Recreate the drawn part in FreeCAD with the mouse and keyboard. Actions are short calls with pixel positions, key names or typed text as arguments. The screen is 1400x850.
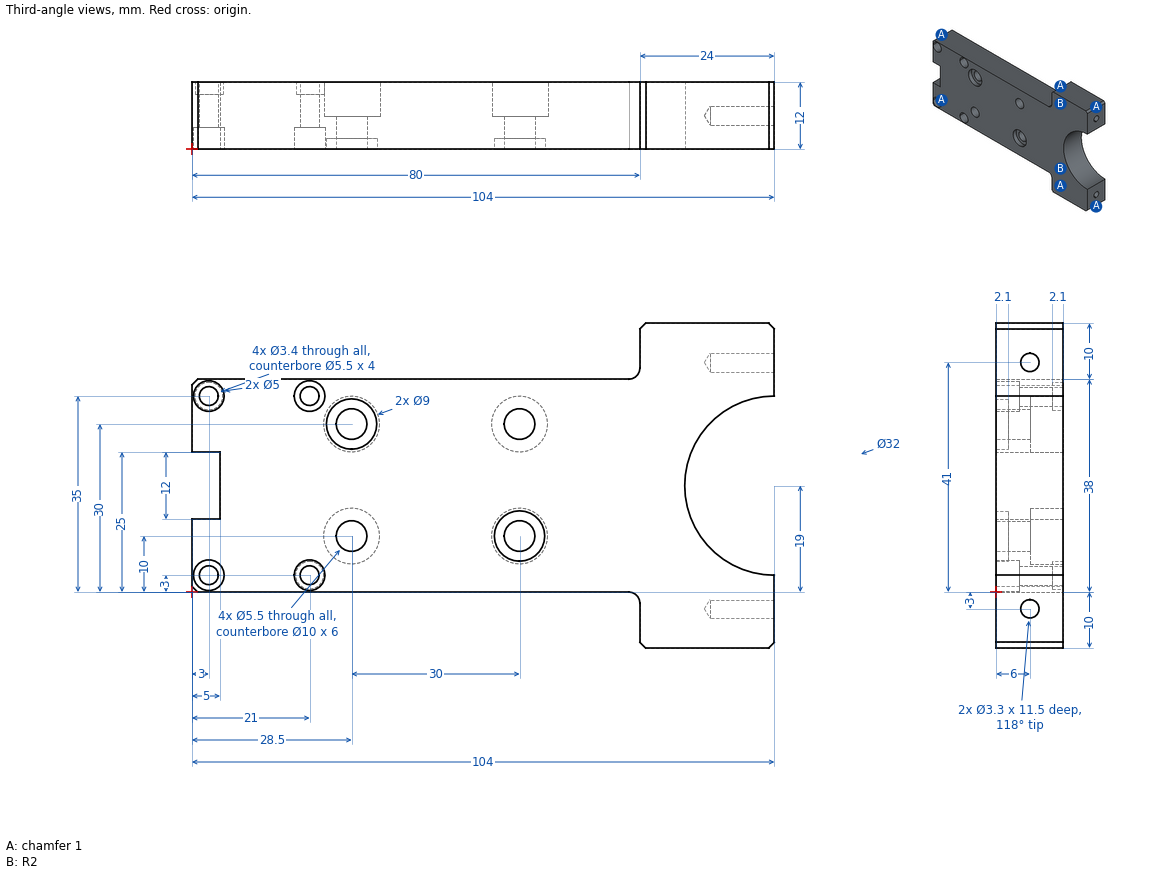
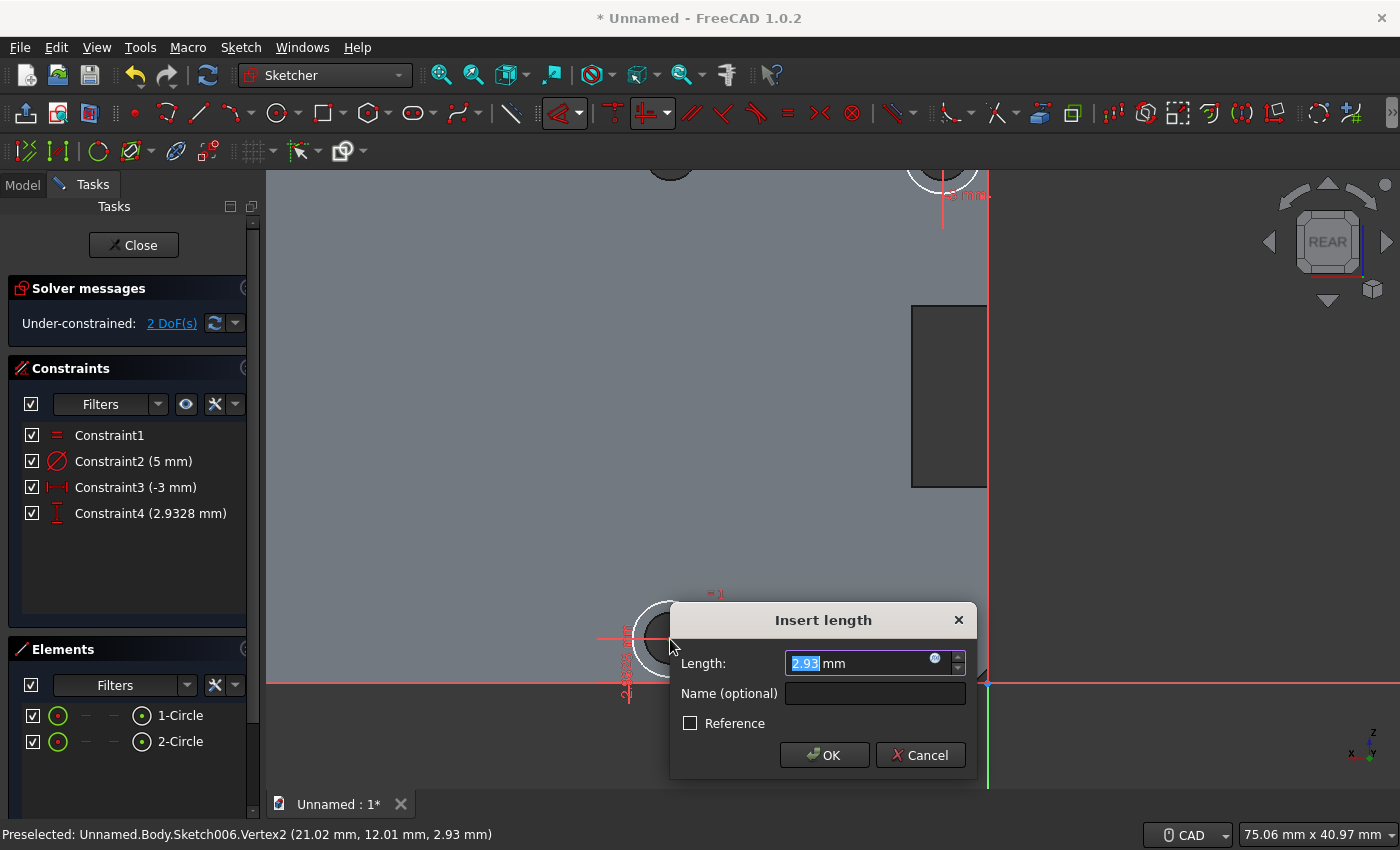
text(3)
key(Return)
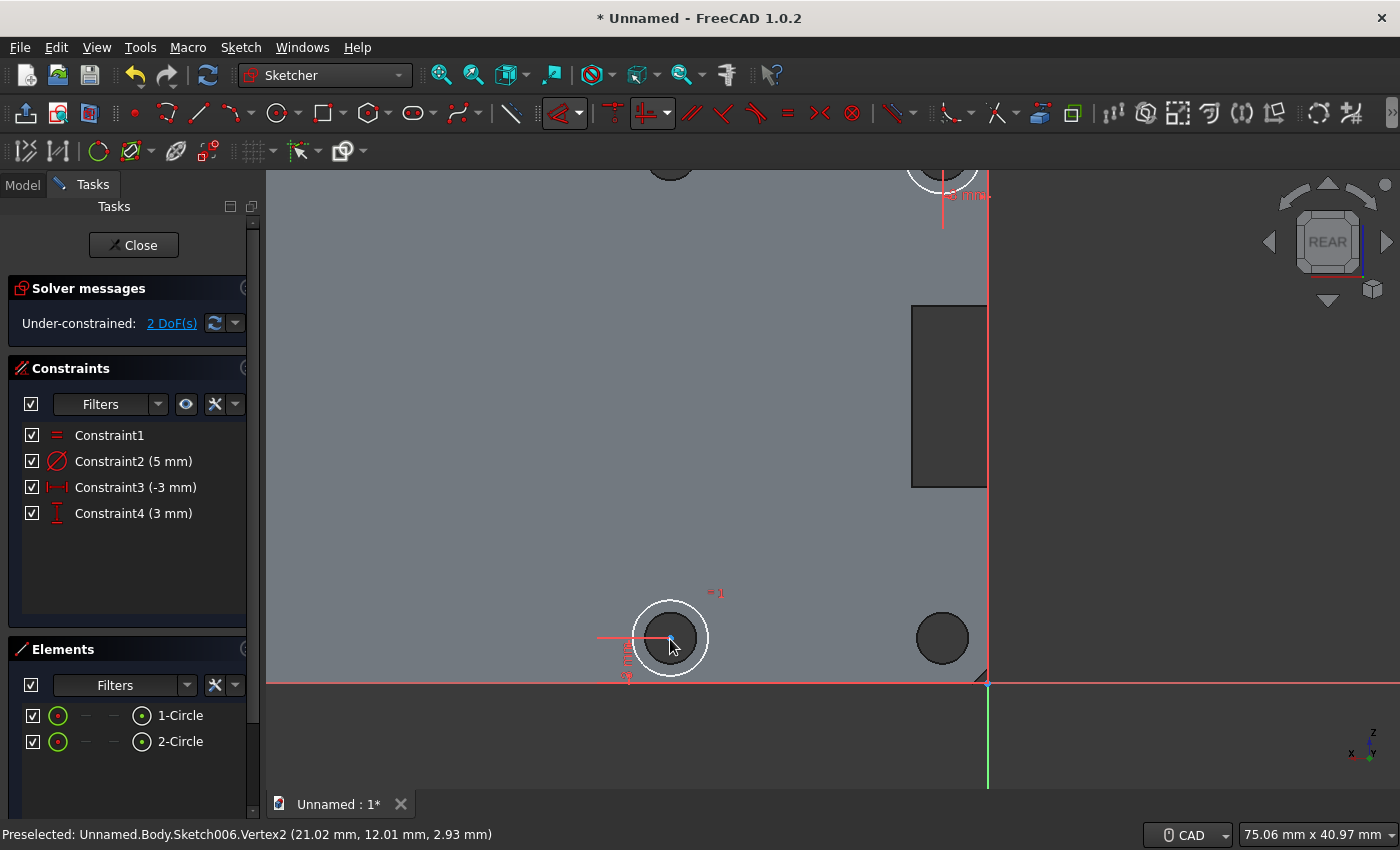
scroll(671, 641, down, 2)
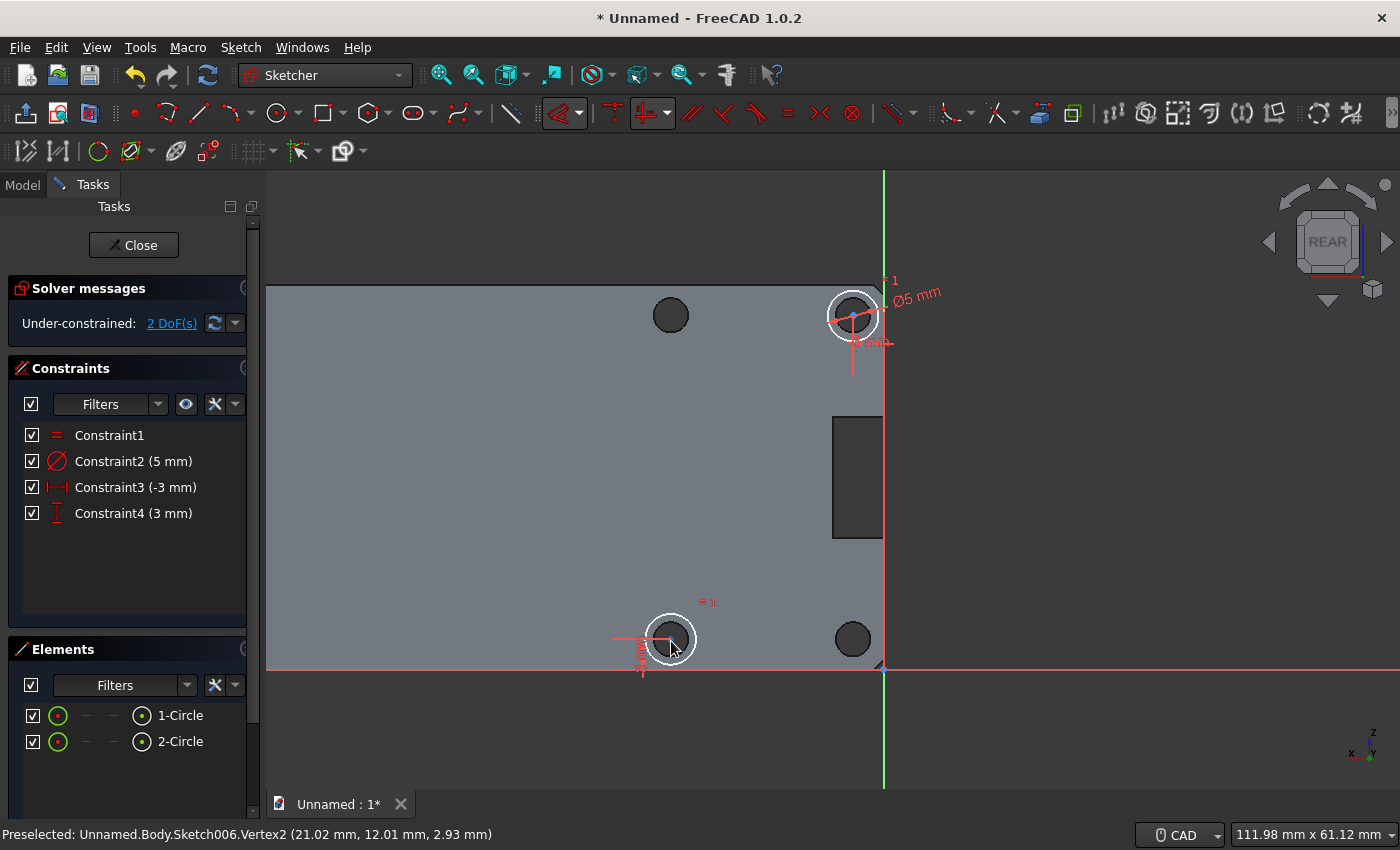
click(853, 316)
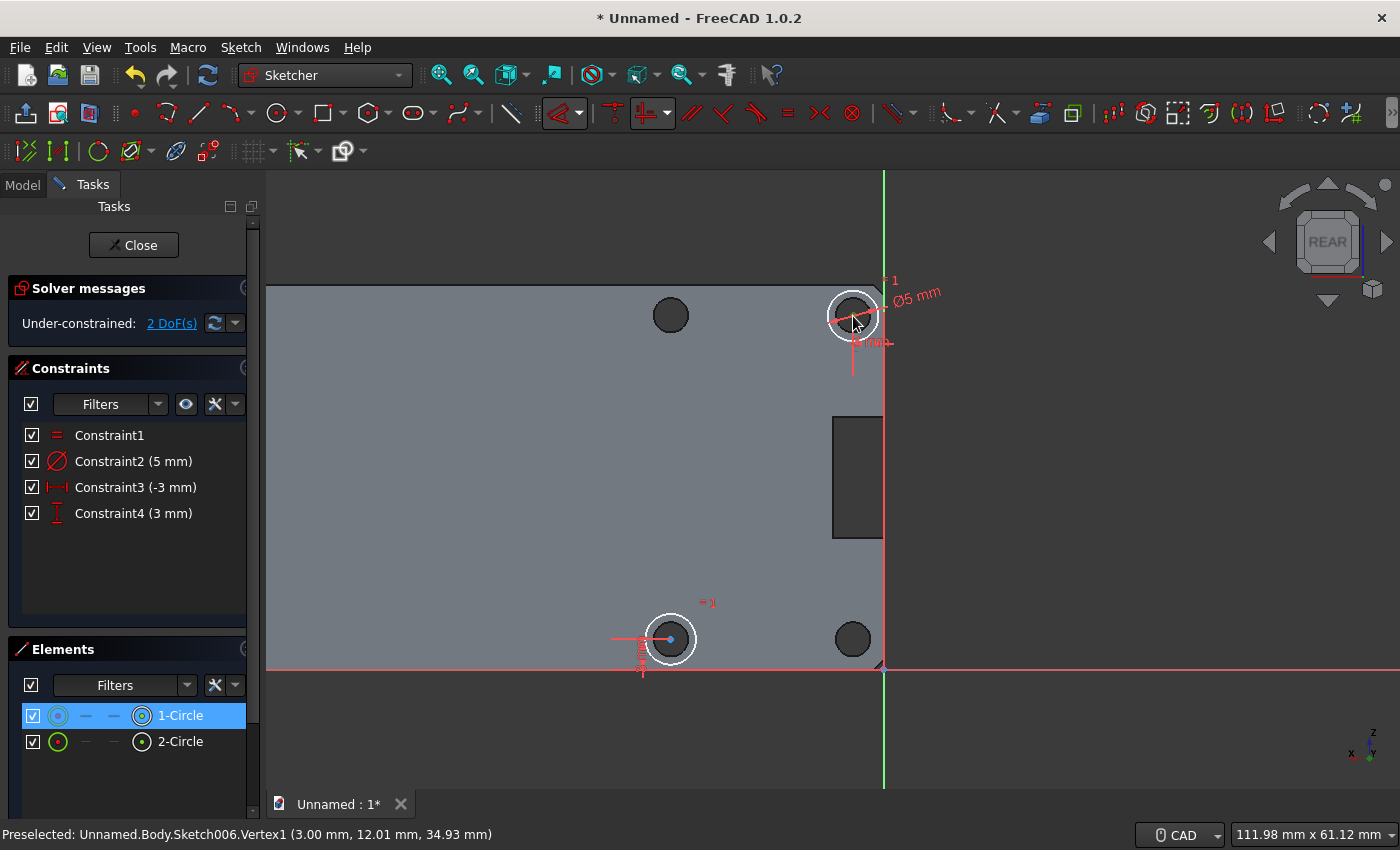
key(i)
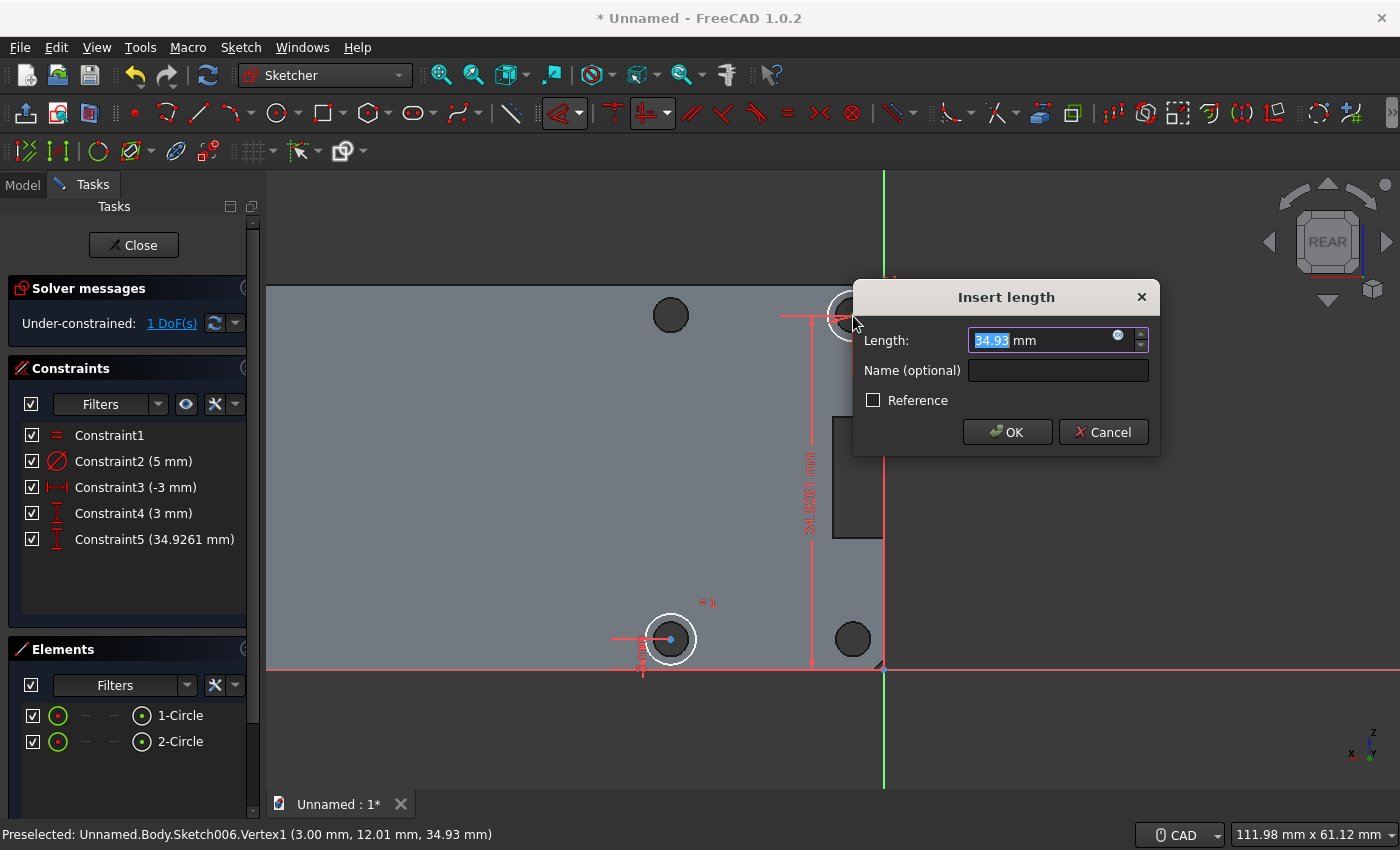
text(35)
key(Return)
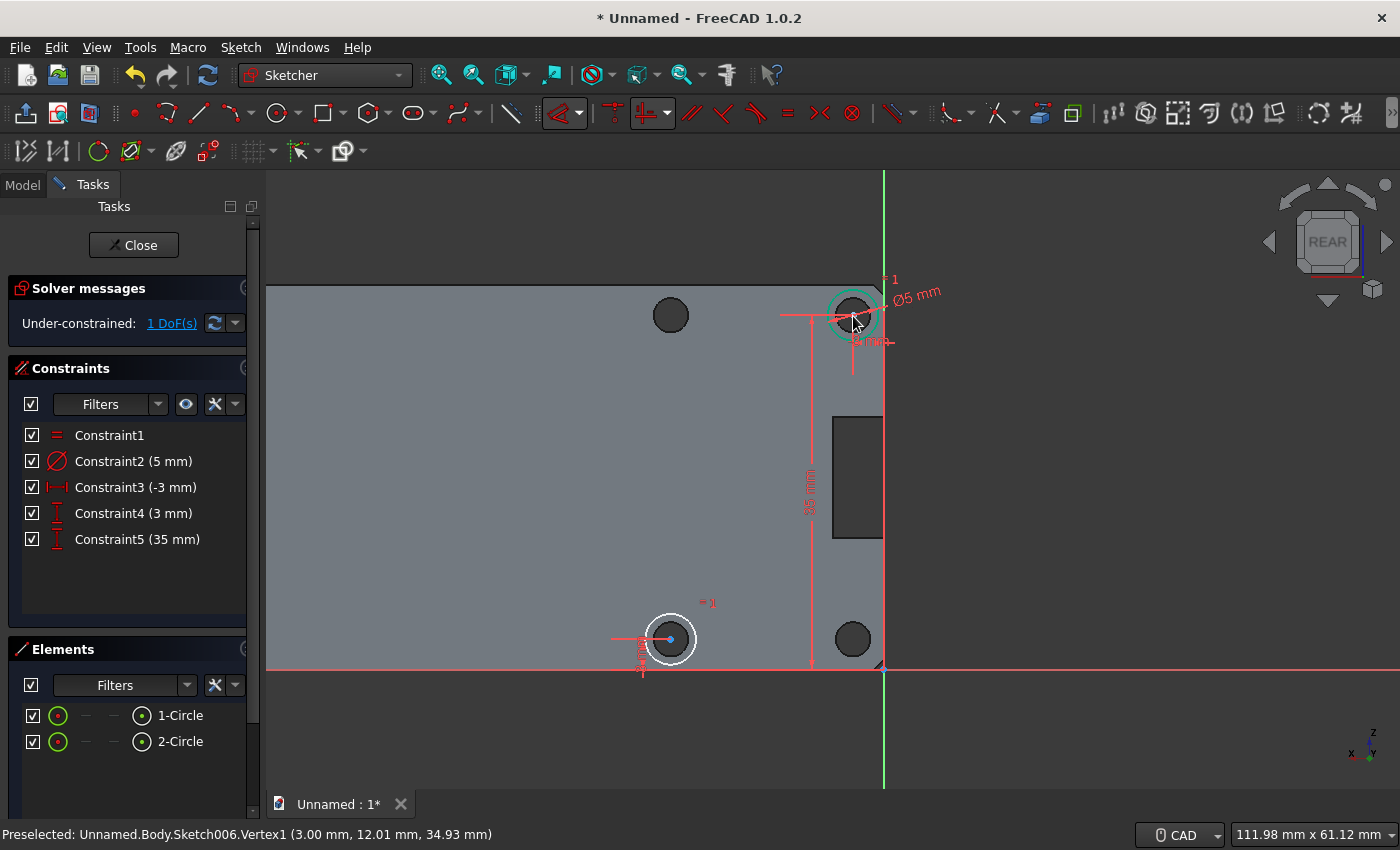
click(671, 639)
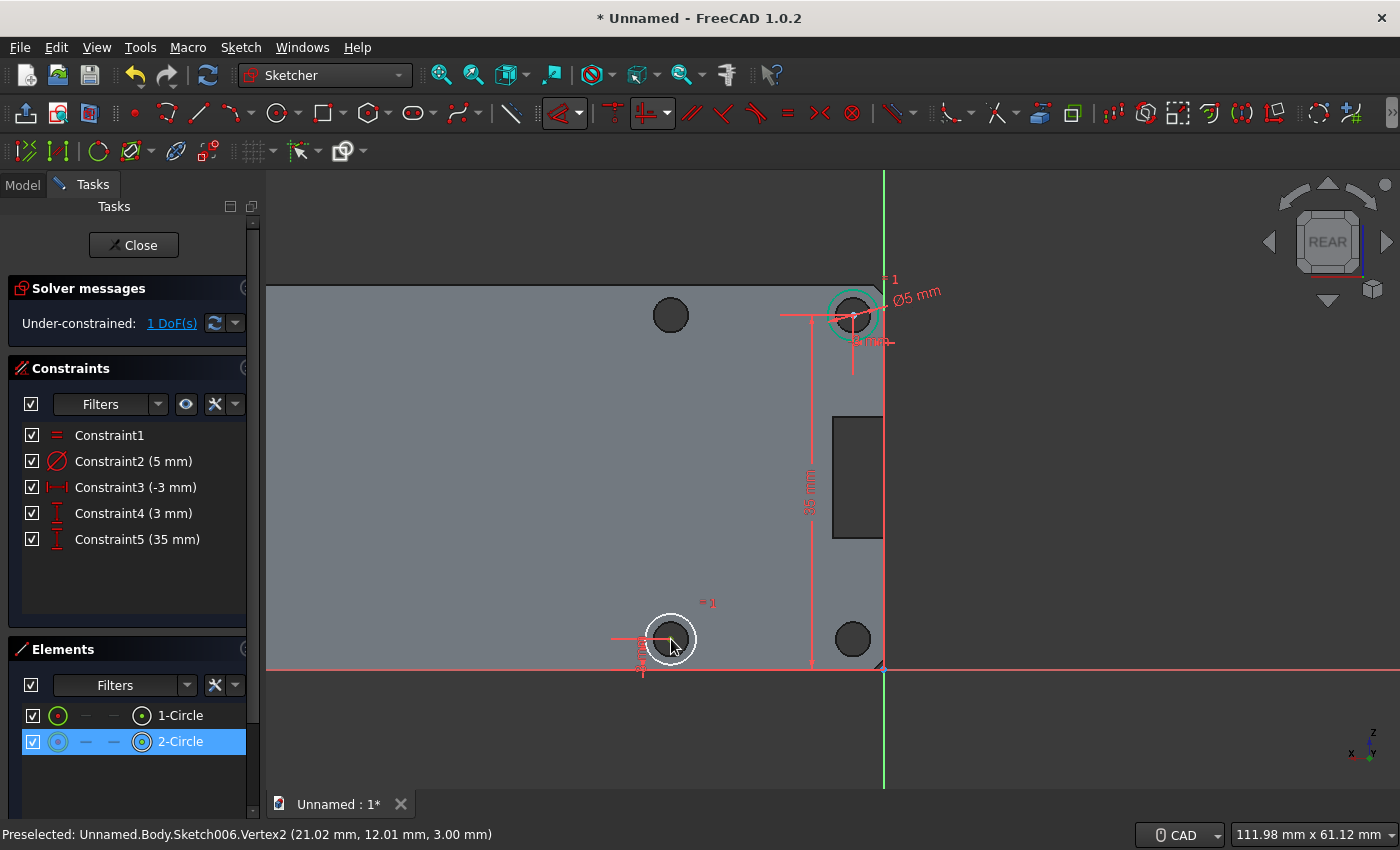
click(582, 114)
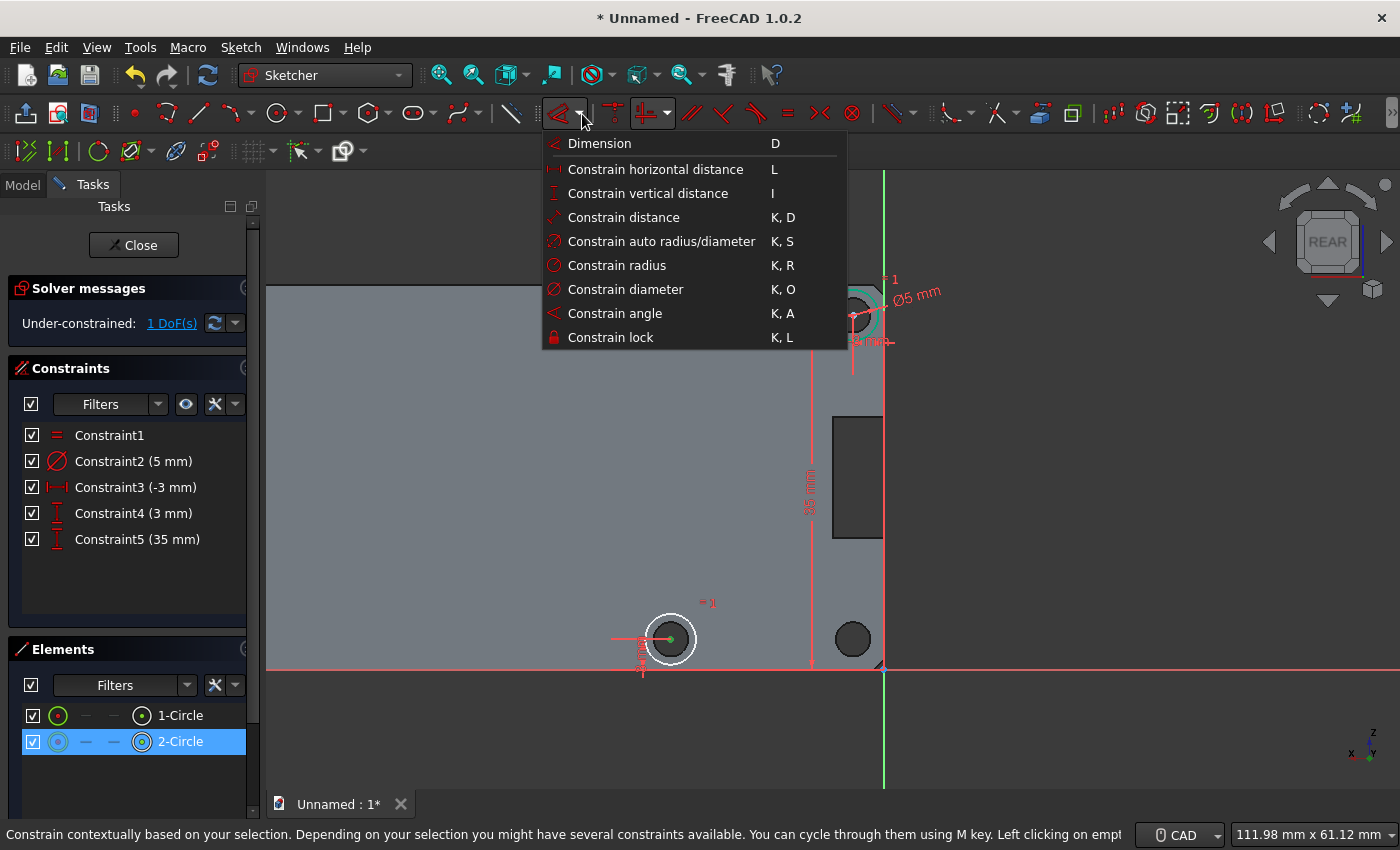
click(695, 169)